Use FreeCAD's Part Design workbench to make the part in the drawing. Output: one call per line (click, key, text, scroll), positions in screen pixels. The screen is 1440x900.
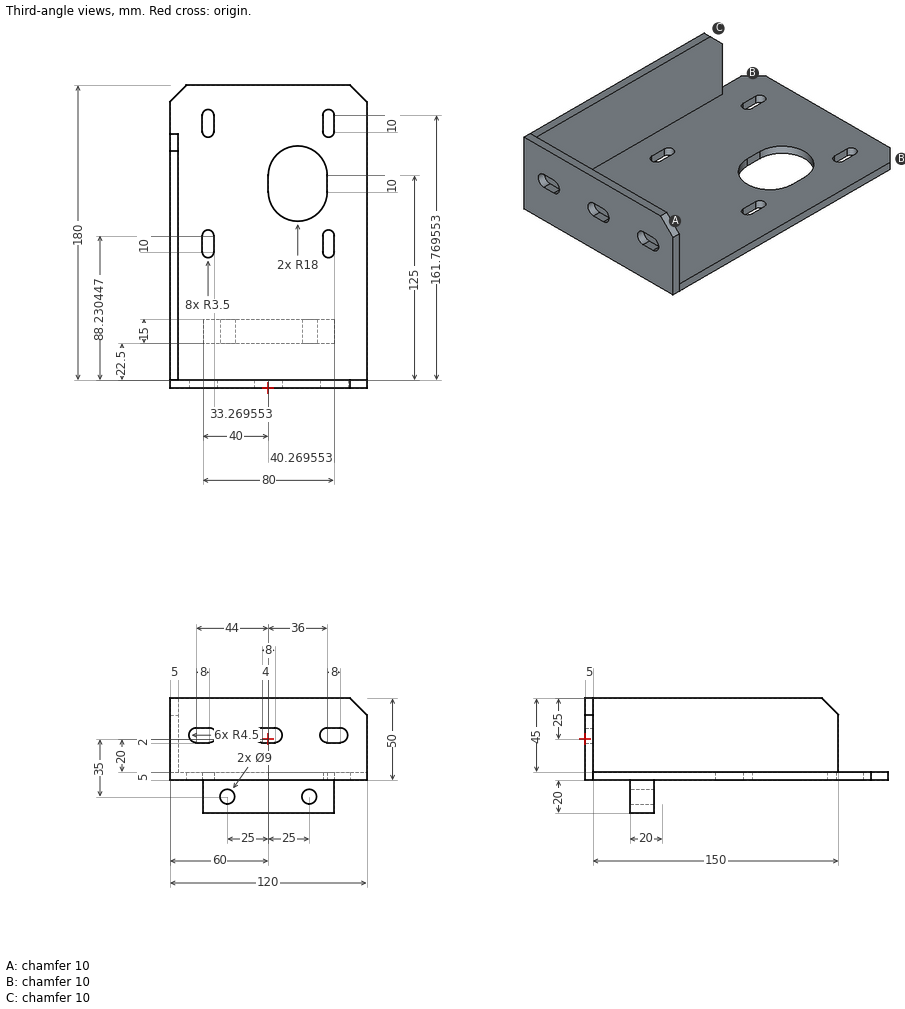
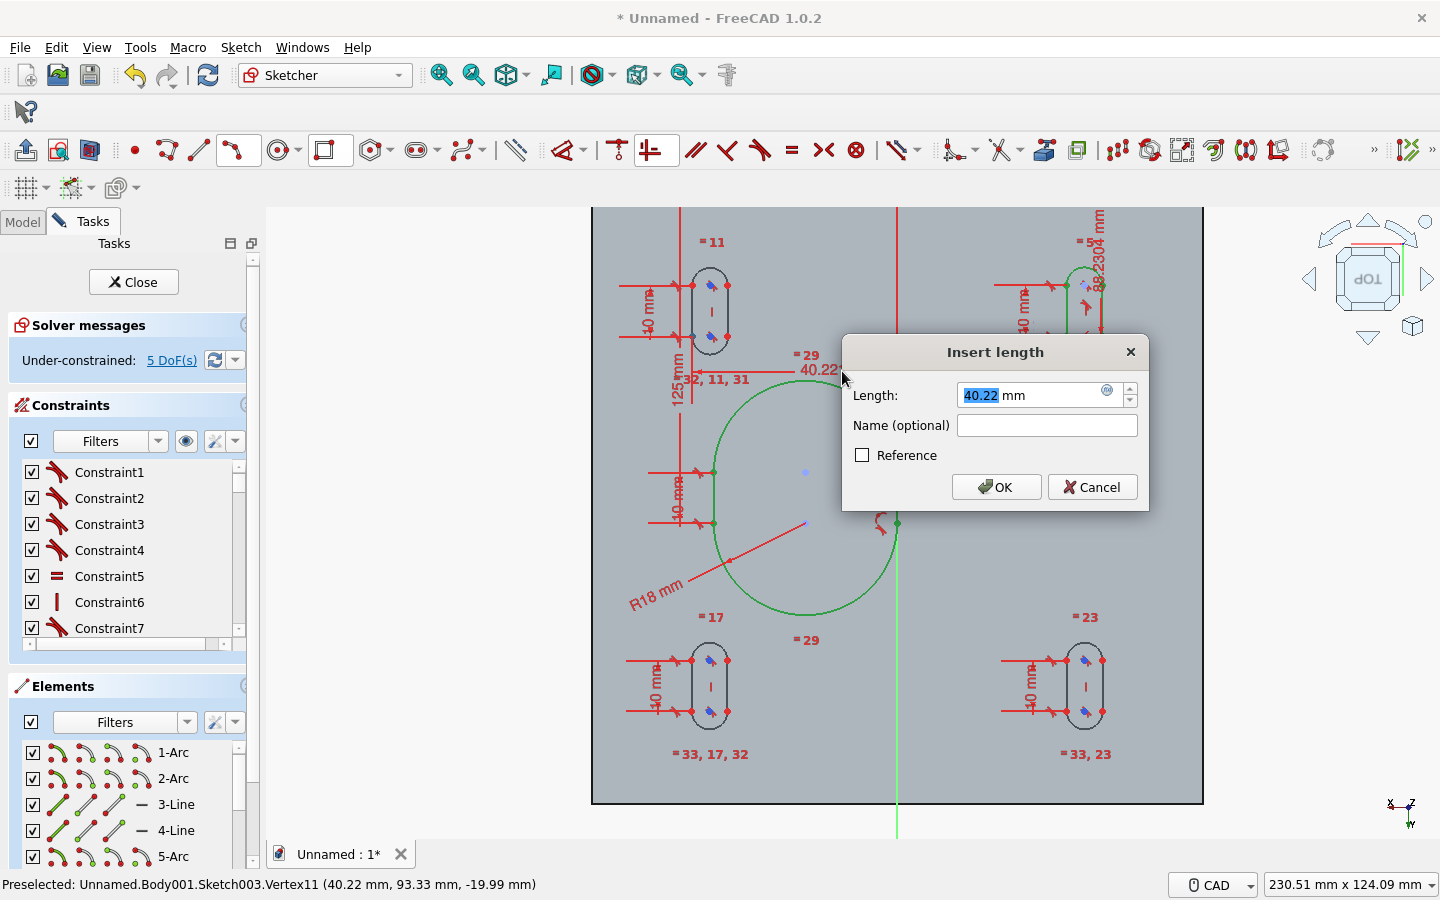
text(40.269553)
key(Return)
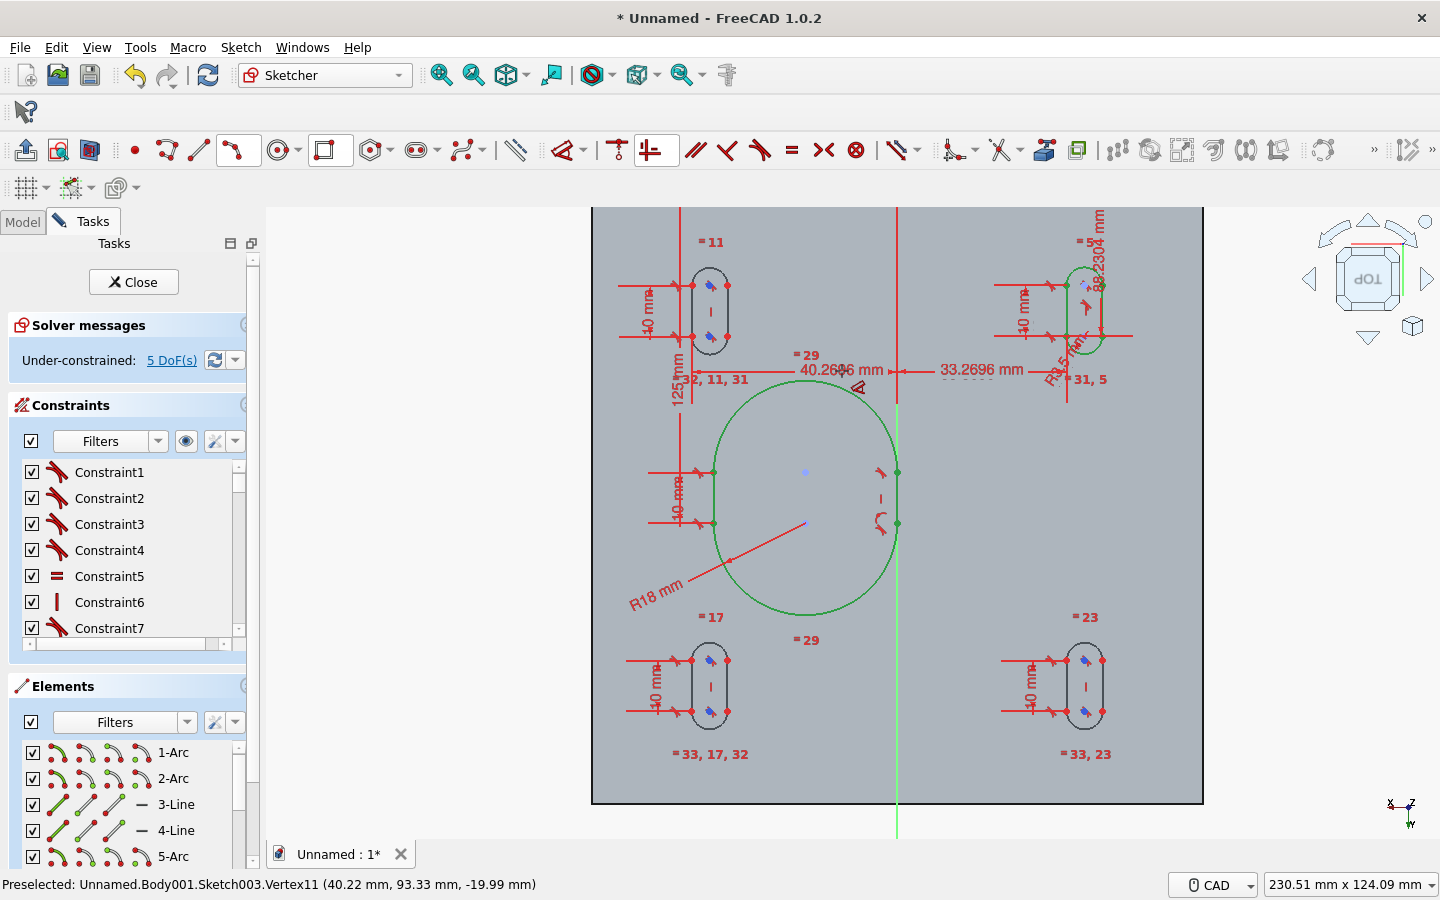
click(692, 337)
click(658, 286)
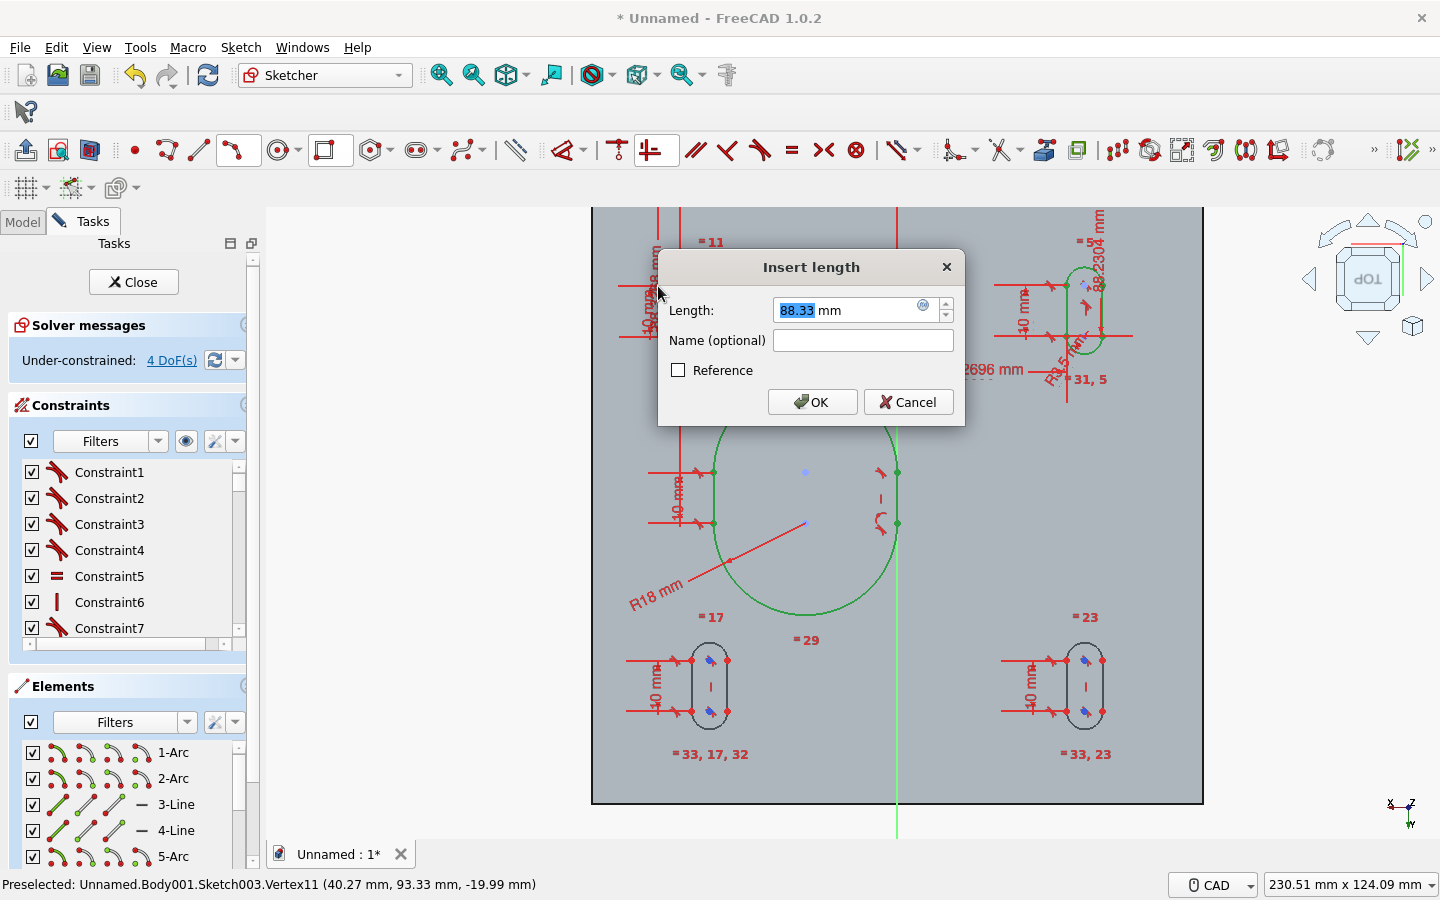
text(88.230447)
key(Return)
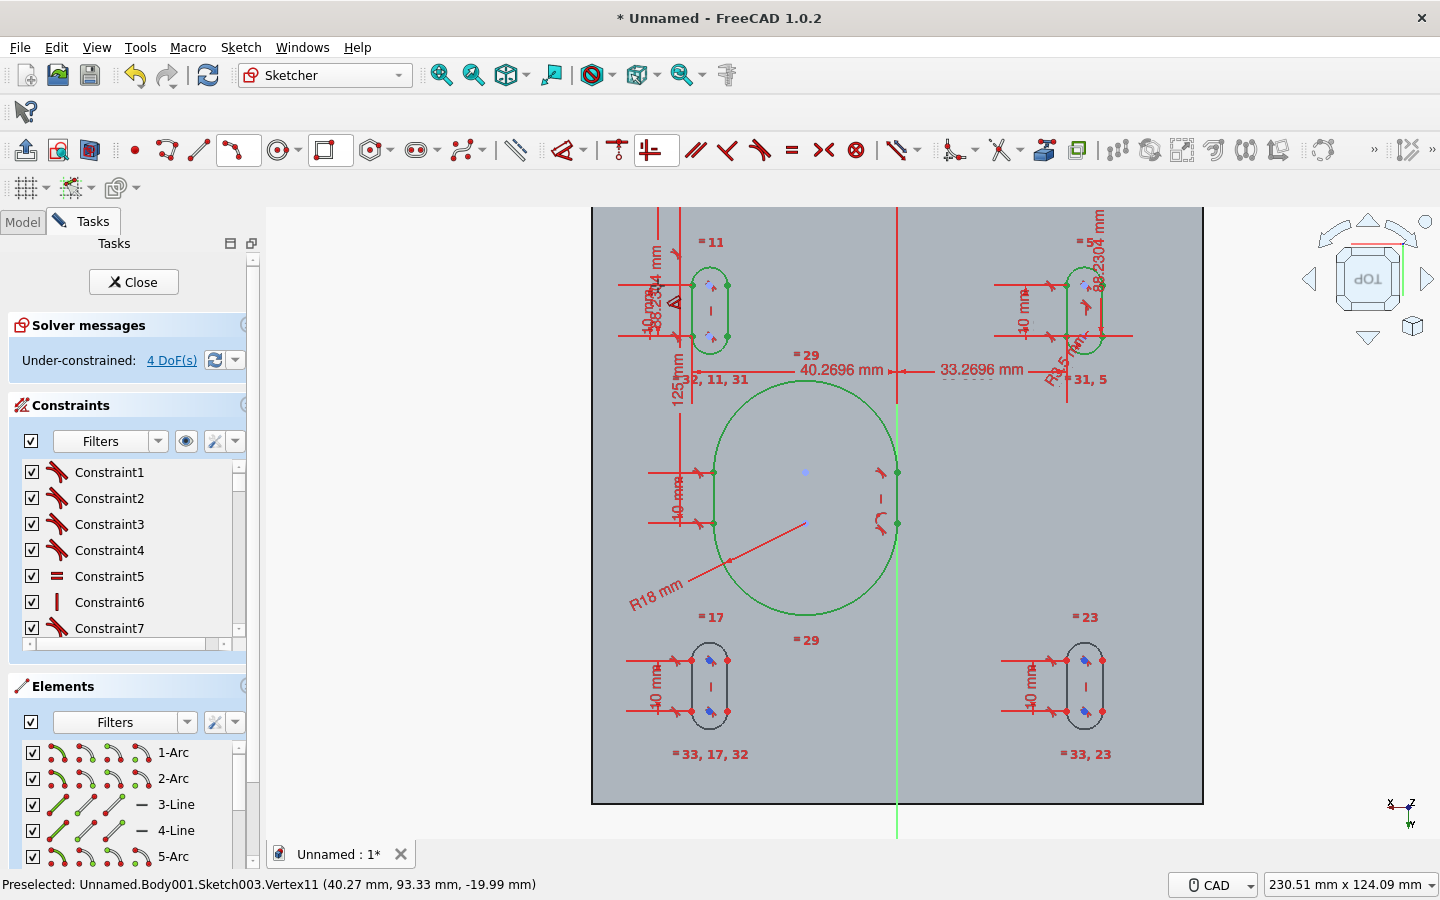
click(692, 711)
click(794, 745)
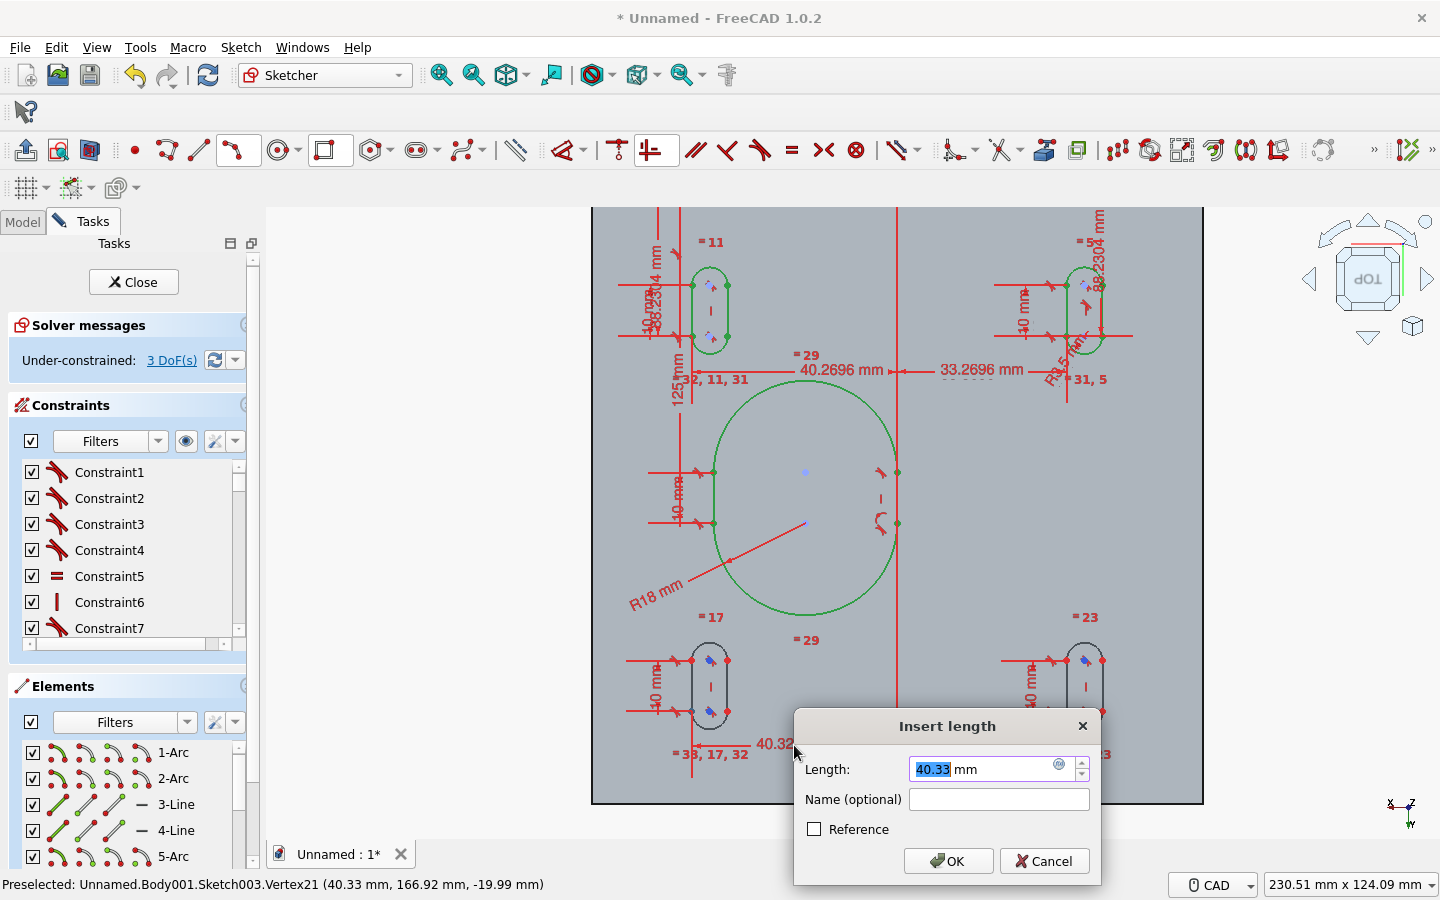
text(40.269553)
key(Return)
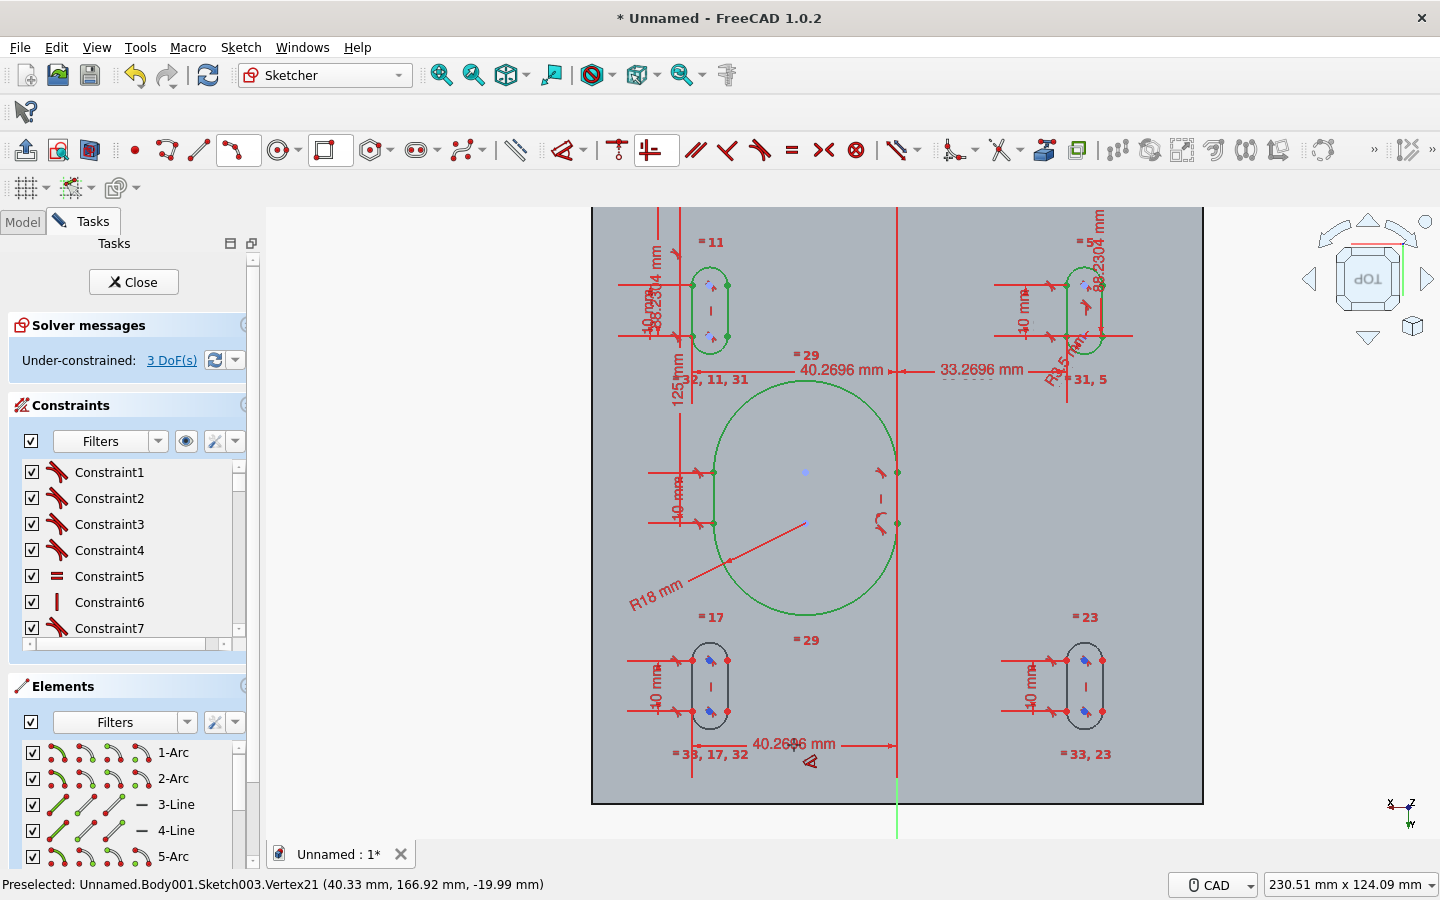
click(1067, 711)
click(982, 745)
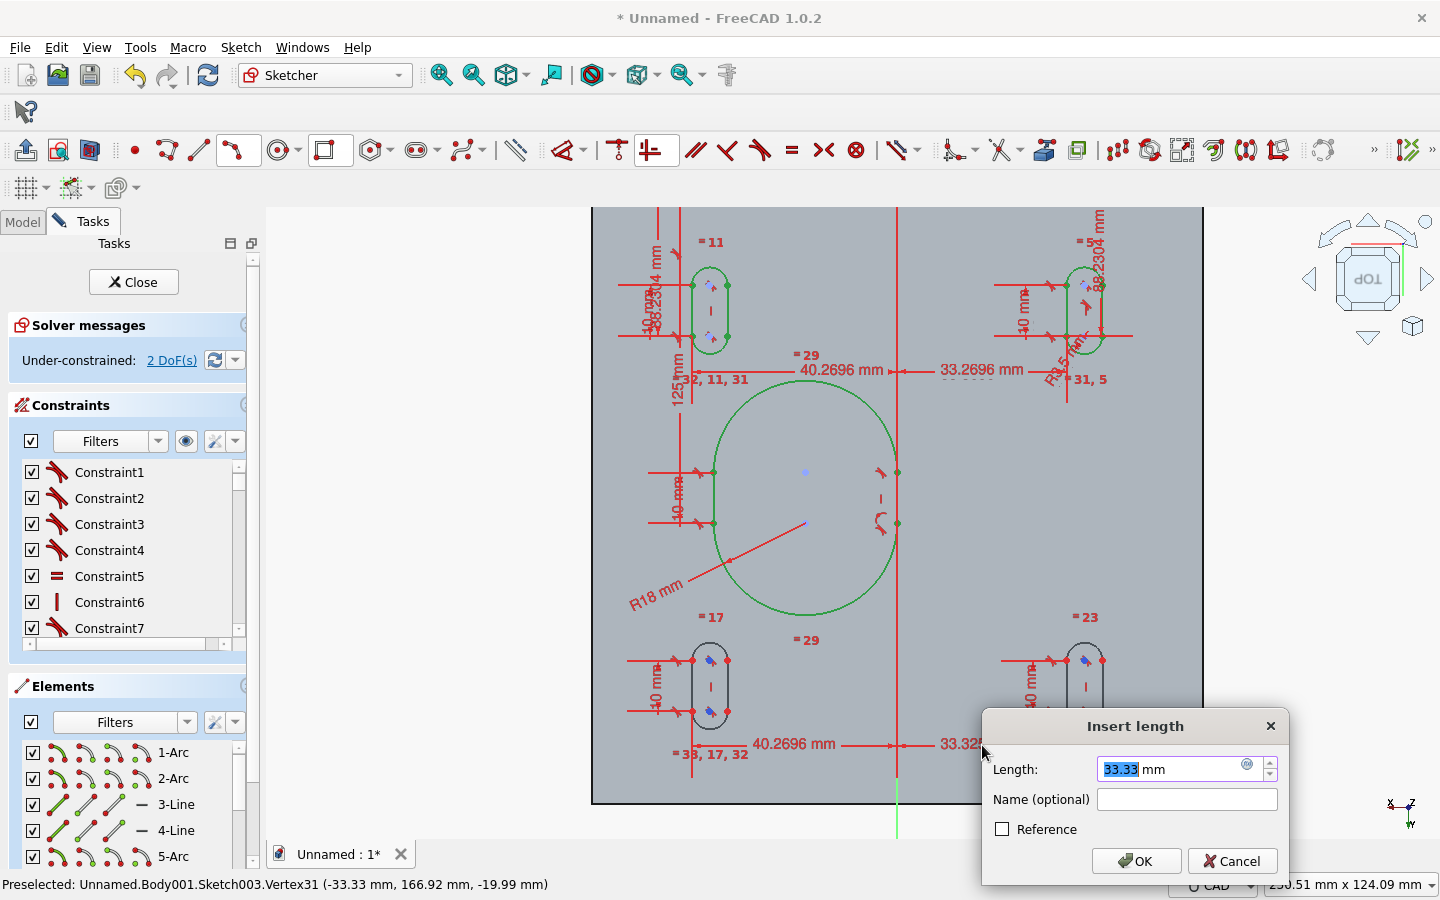
text(33.269553)
key(Return)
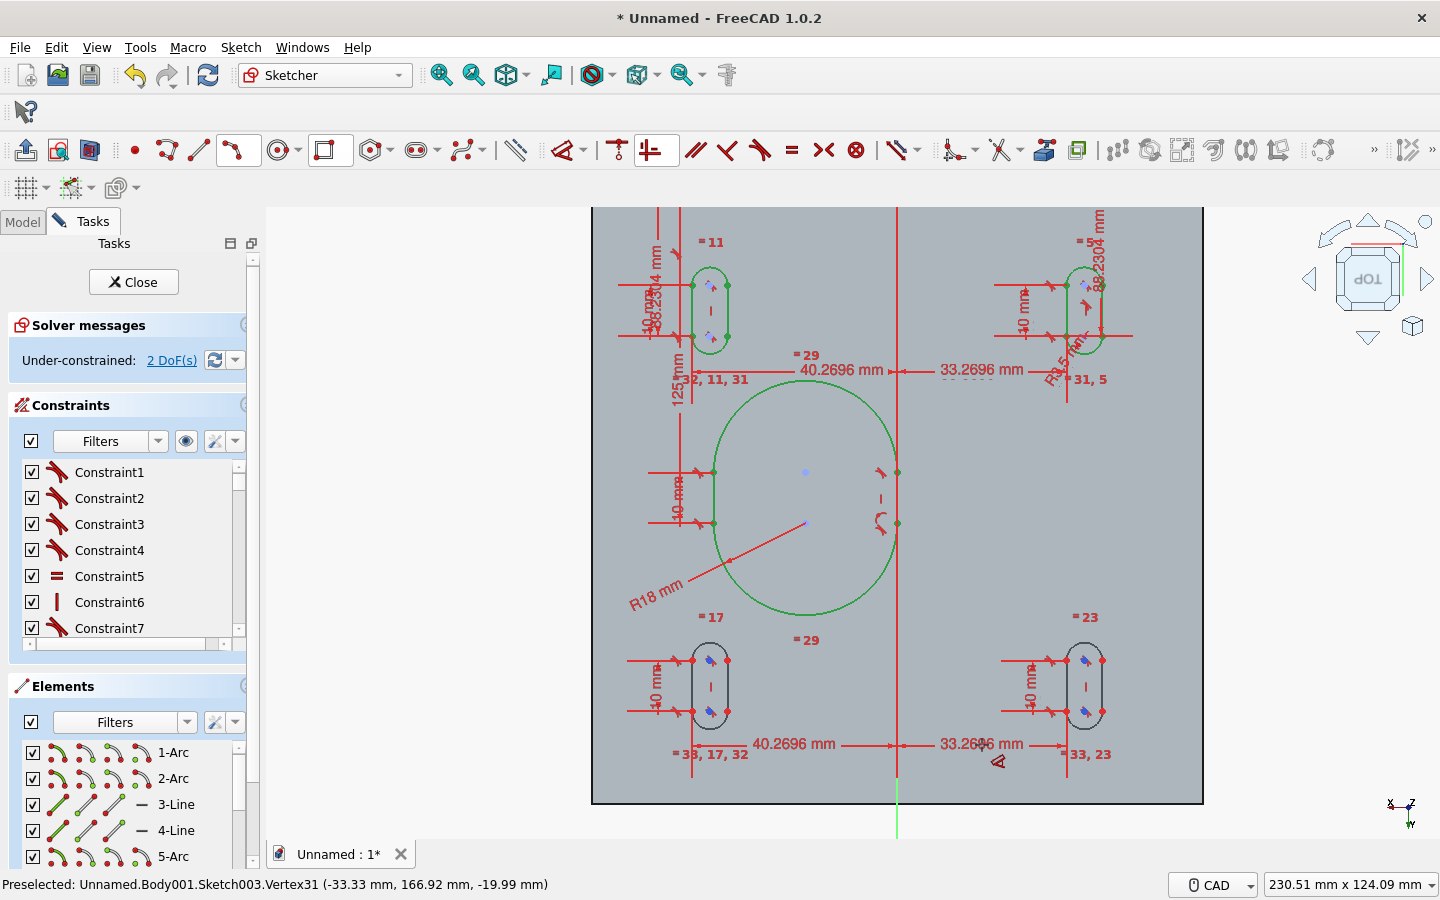
click(692, 711)
click(658, 473)